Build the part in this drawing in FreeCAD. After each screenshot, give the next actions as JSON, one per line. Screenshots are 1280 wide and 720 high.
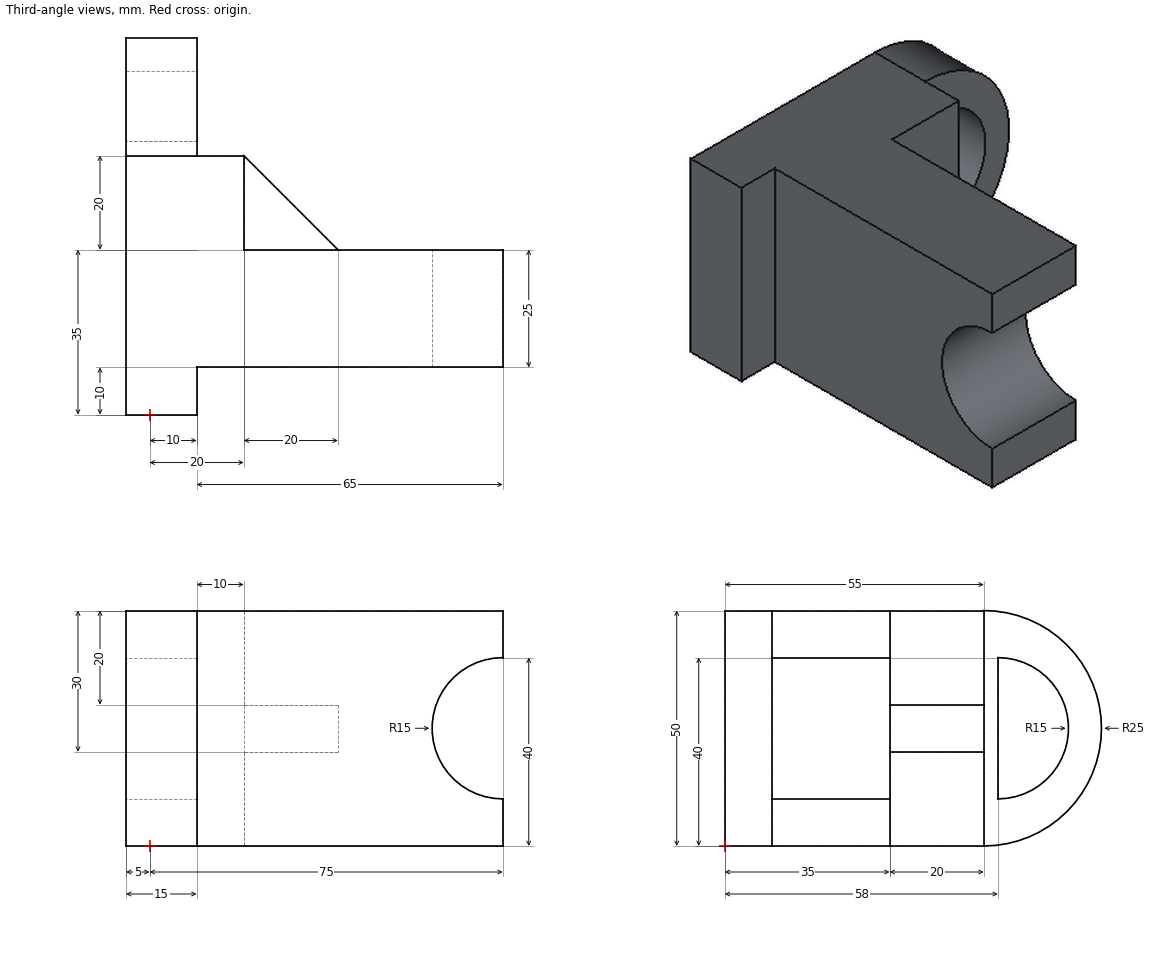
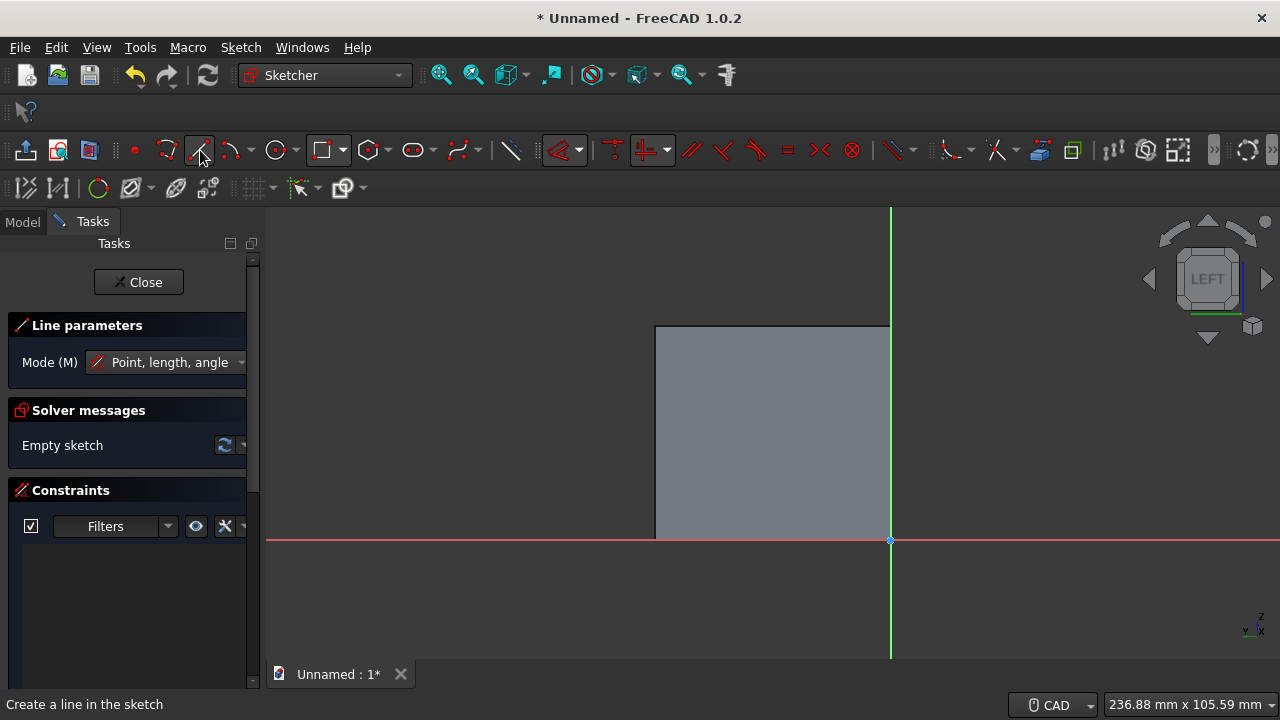
{"action": "left_click", "coordinate": [655, 540]}
{"action": "left_click", "coordinate": [655, 326]}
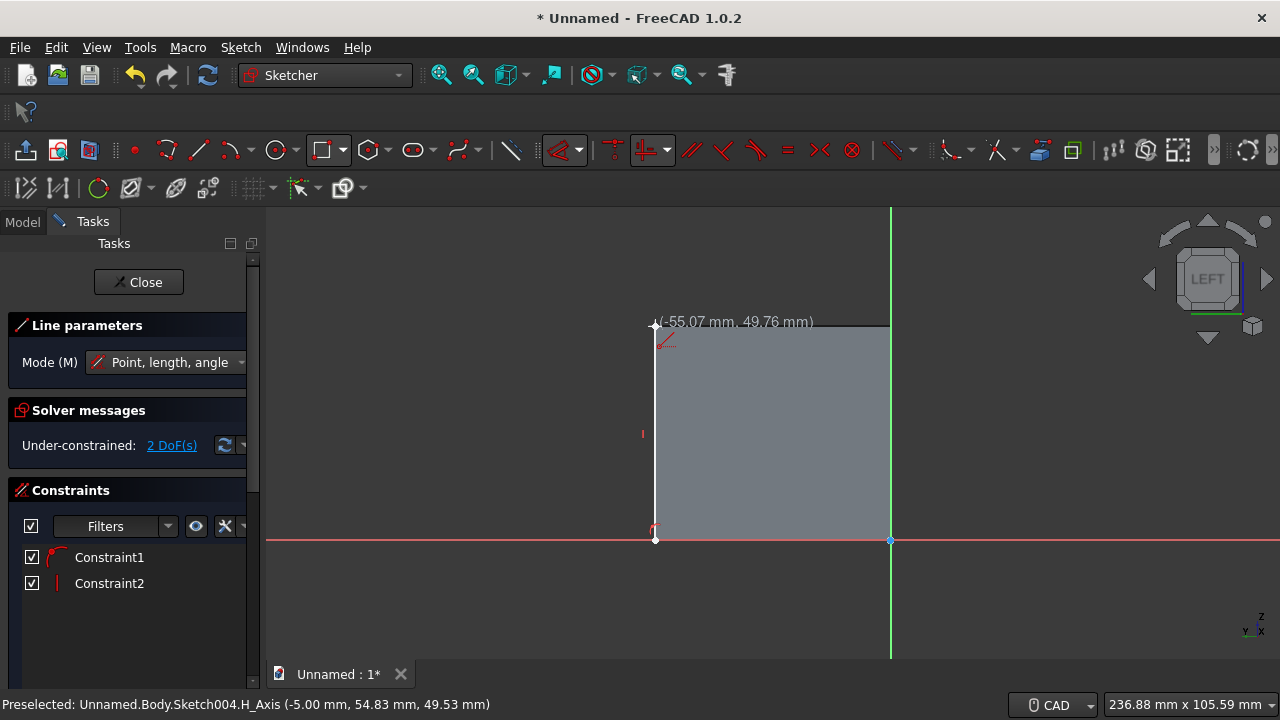
{"action": "left_click", "coordinate": [254, 150]}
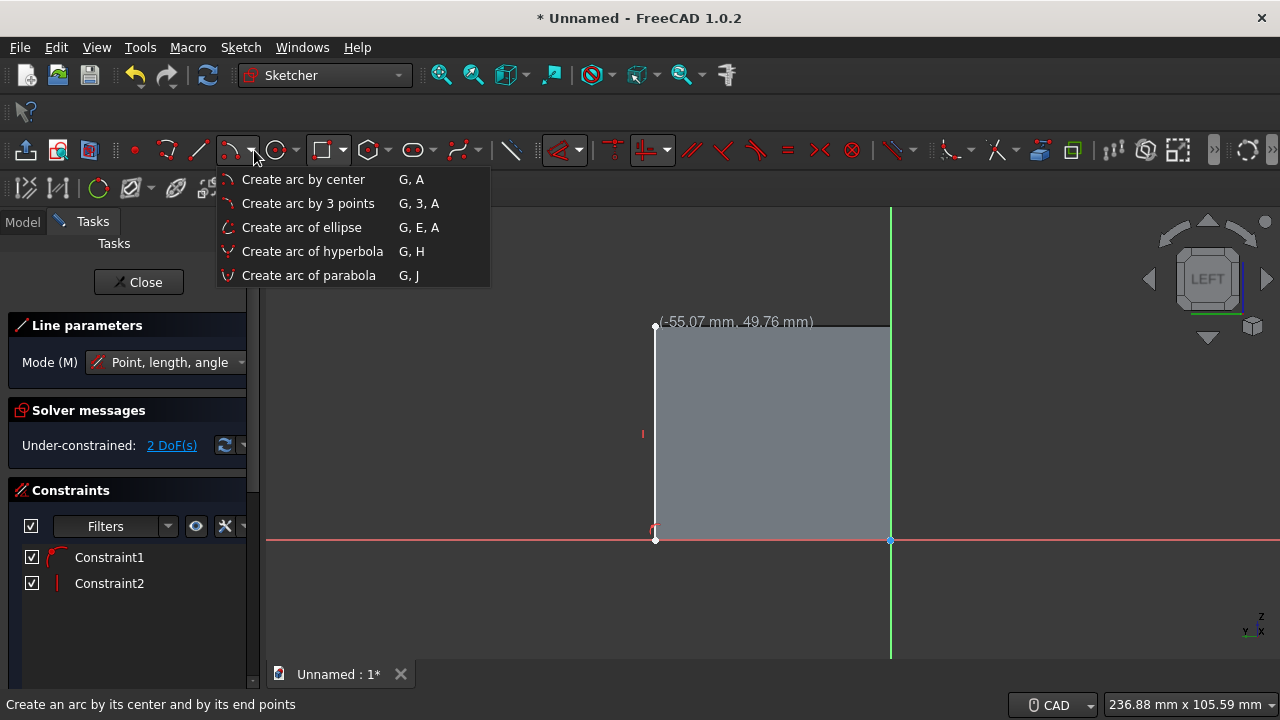
{"action": "left_click", "coordinate": [354, 203]}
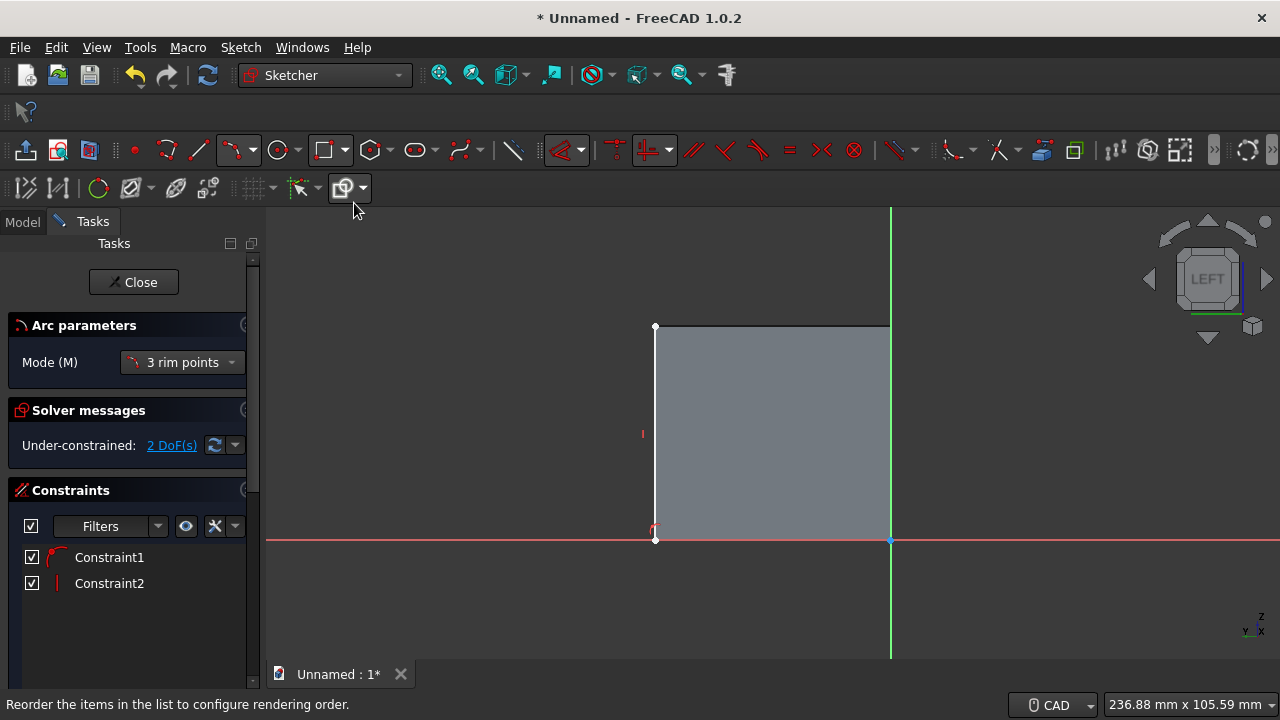
{"action": "left_click", "coordinate": [655, 327]}
{"action": "left_click", "coordinate": [655, 540]}
{"action": "left_click", "coordinate": [548, 433]}
{"action": "key", "text": "Escape"}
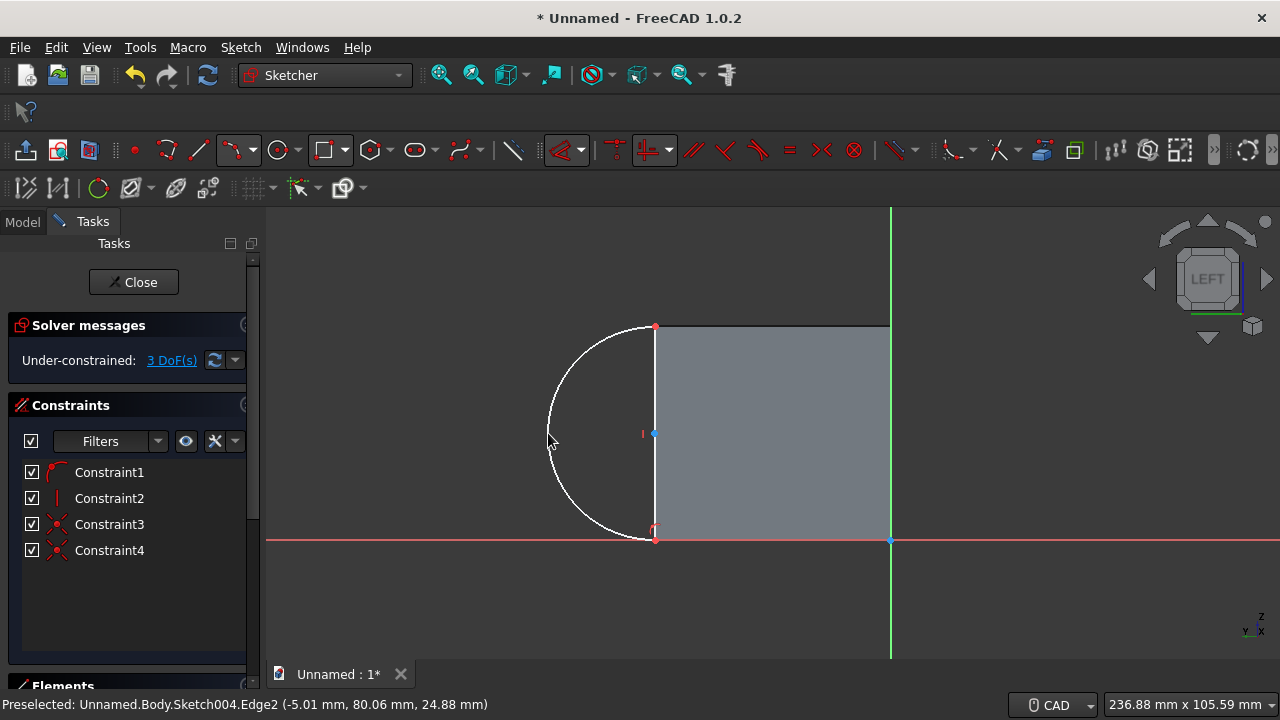
{"action": "left_click", "coordinate": [568, 371]}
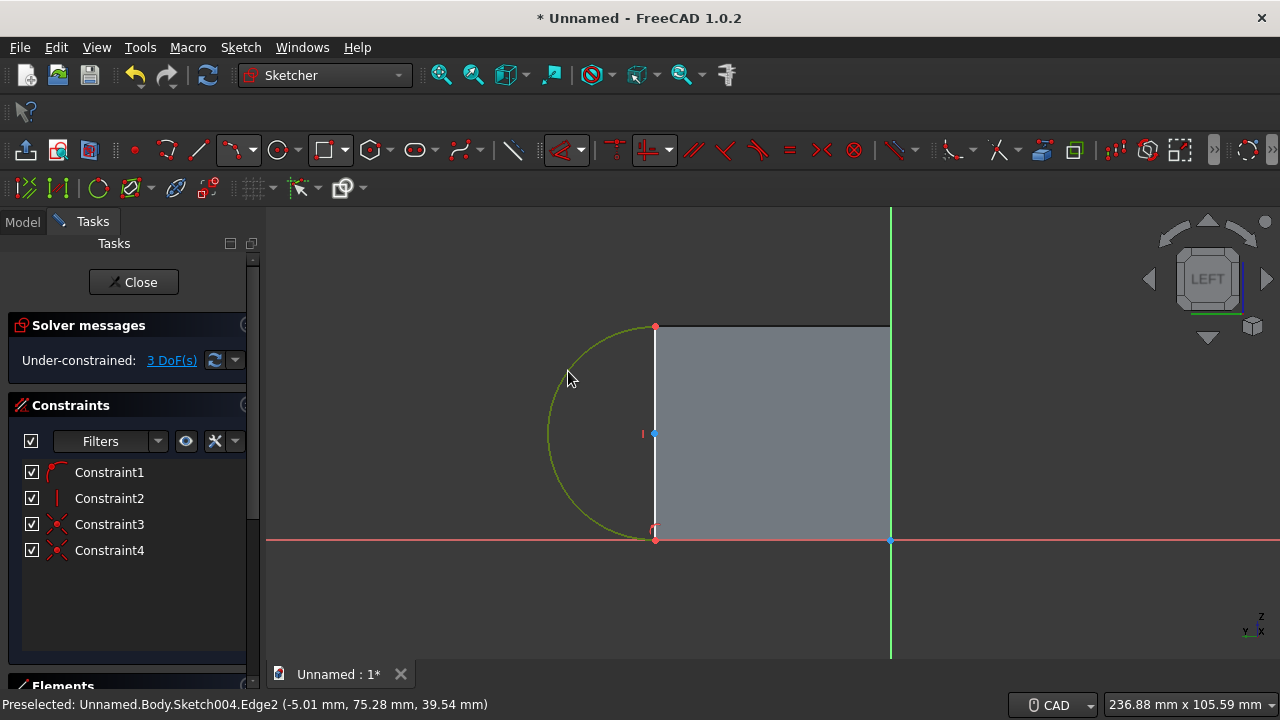
{"action": "key", "text": "k r"}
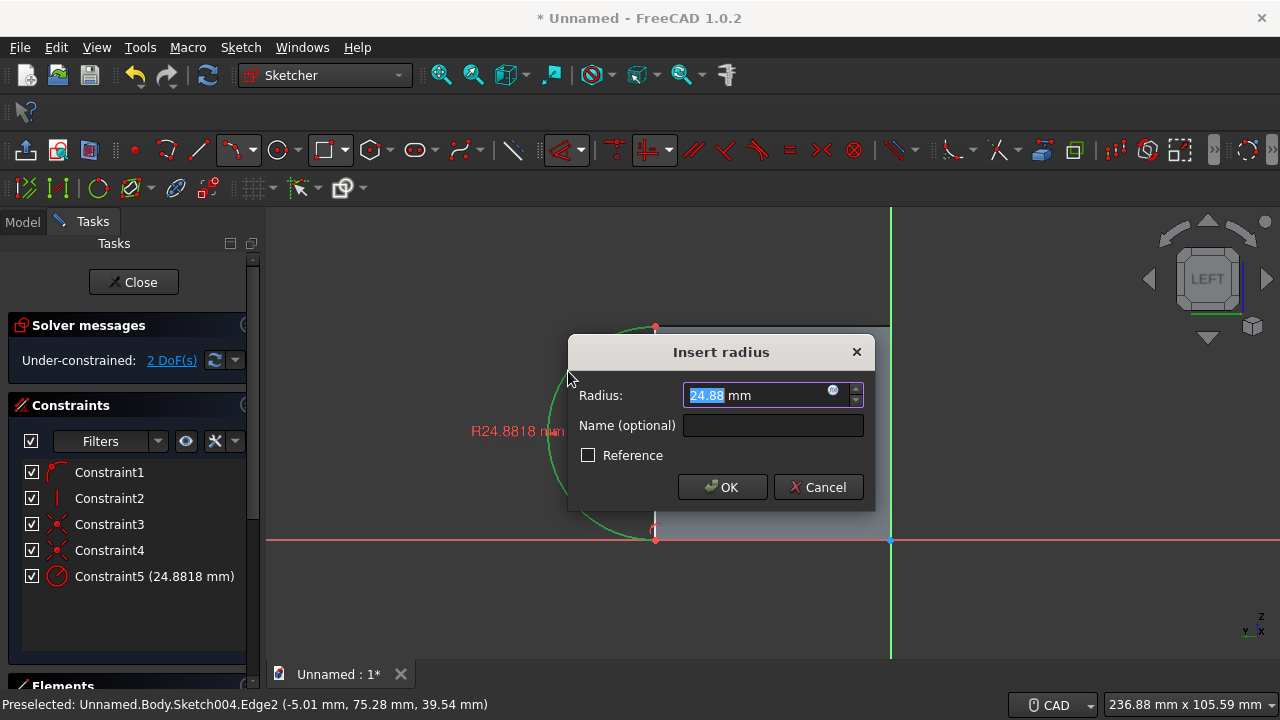
{"action": "type", "text": "25"}
{"action": "key", "text": "Return"}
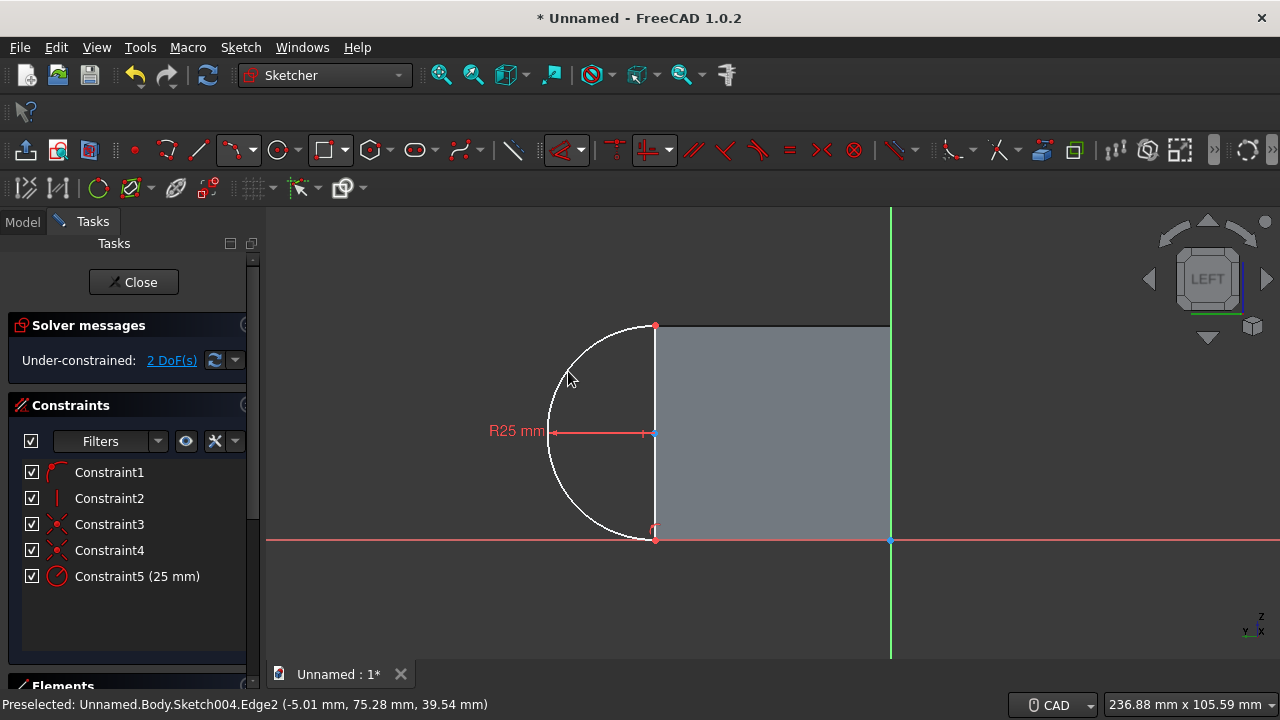
{"action": "left_click", "coordinate": [655, 540]}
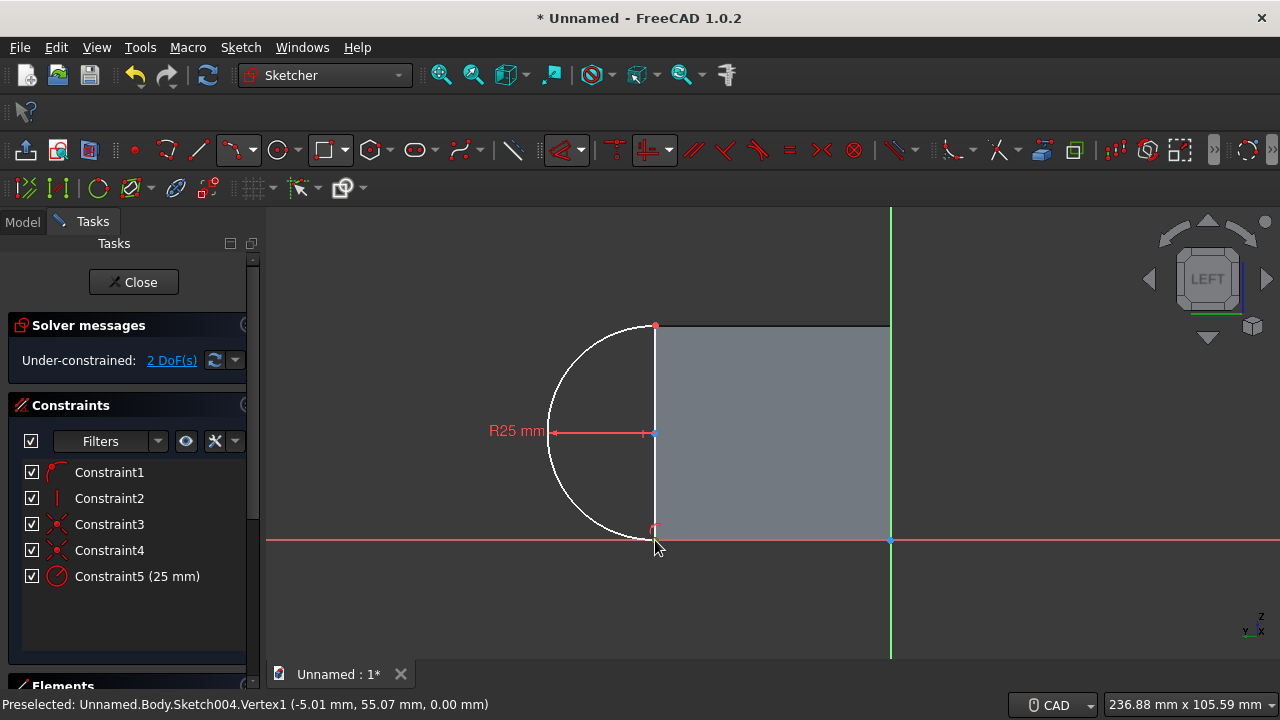
{"action": "left_click", "coordinate": [584, 150]}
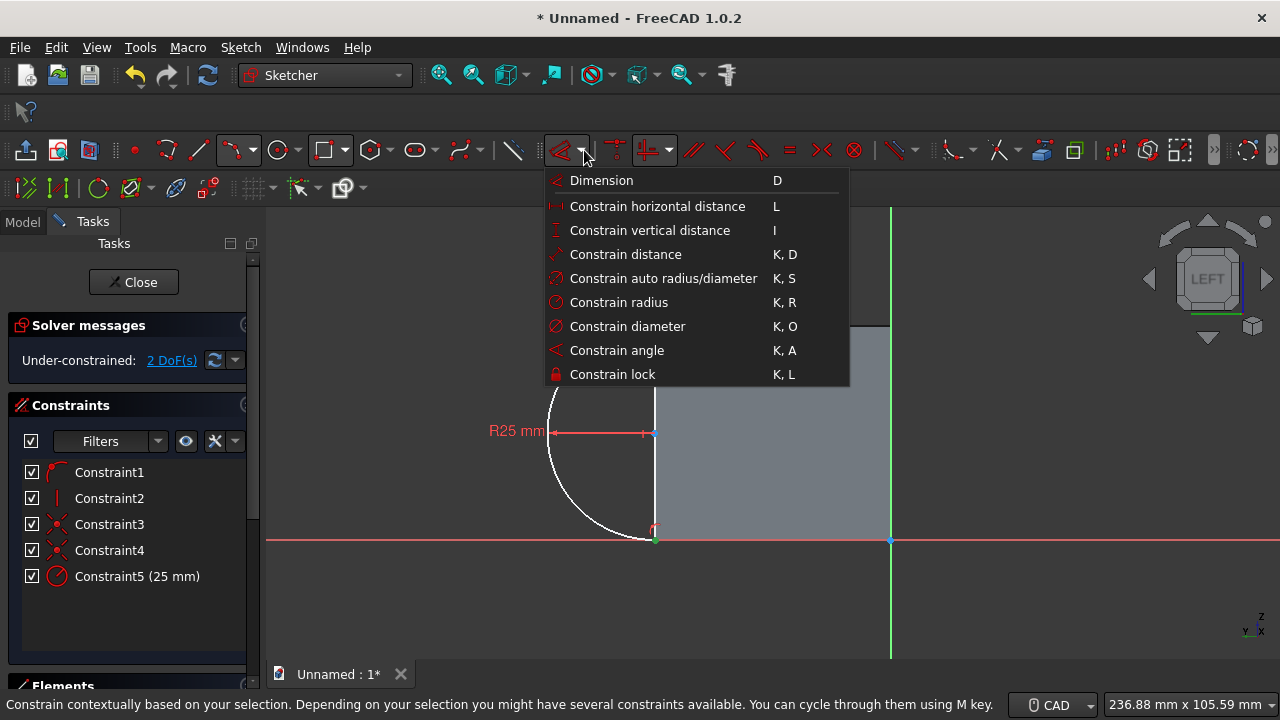
{"action": "left_click", "coordinate": [697, 206]}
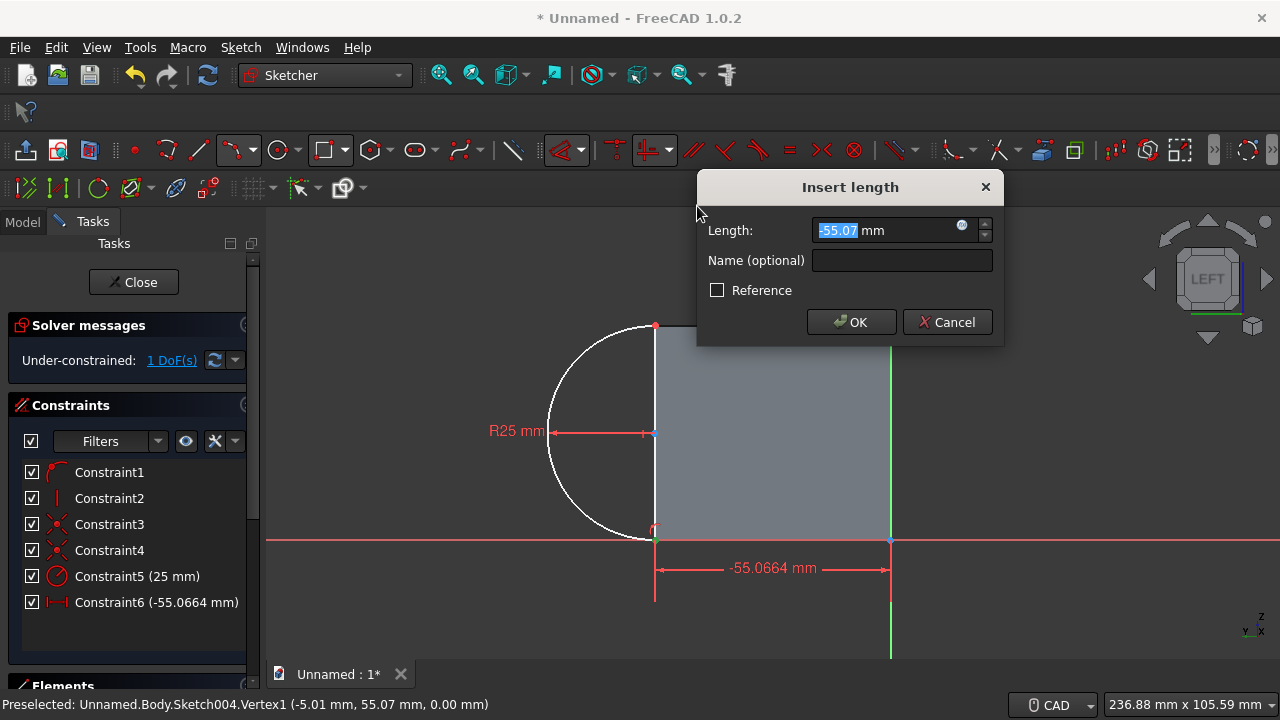
{"action": "type", "text": "-55"}
{"action": "key", "text": "Return"}